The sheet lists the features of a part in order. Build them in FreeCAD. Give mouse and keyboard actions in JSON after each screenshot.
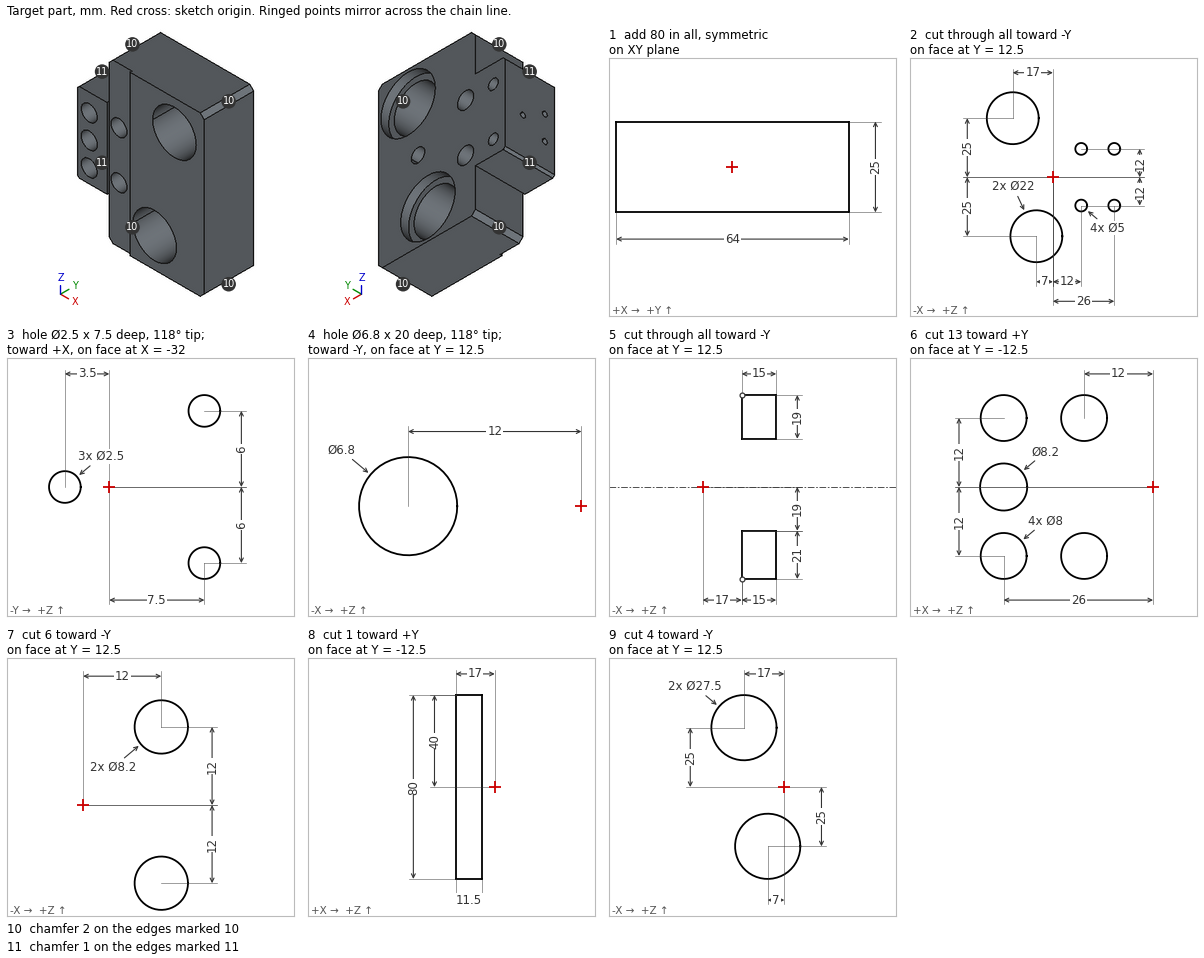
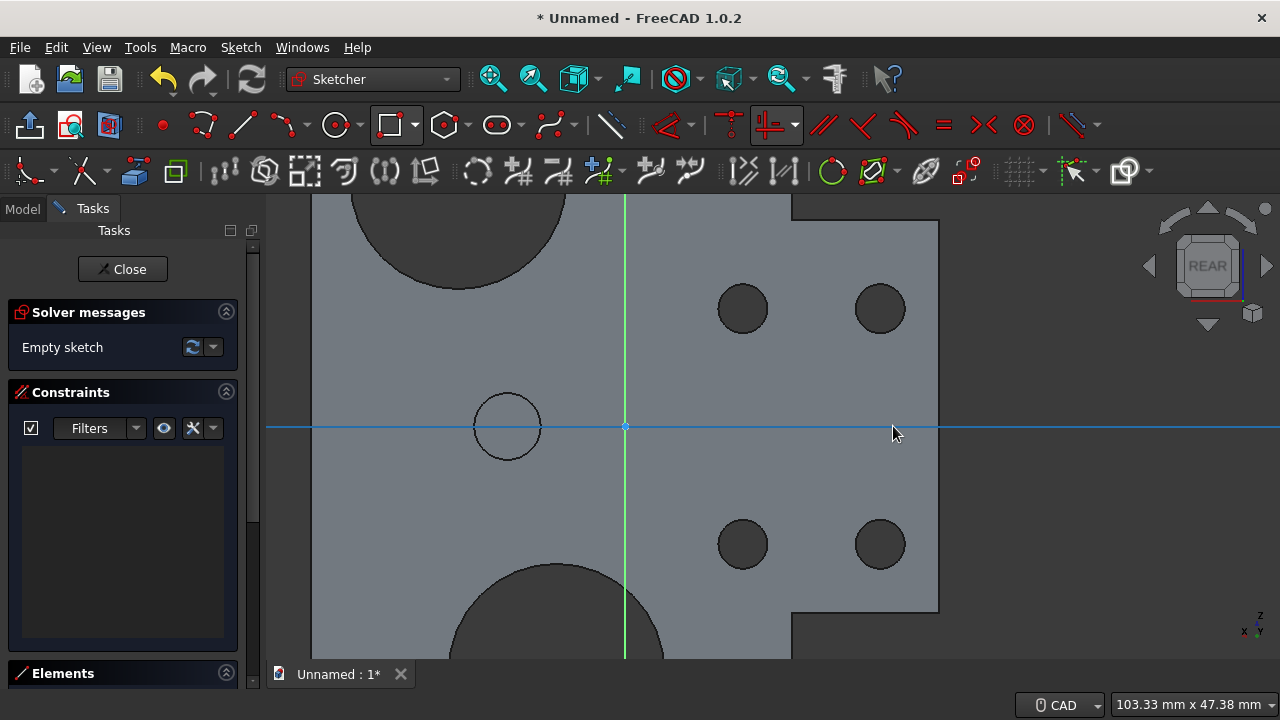
{"action": "left_click", "coordinate": [336, 126]}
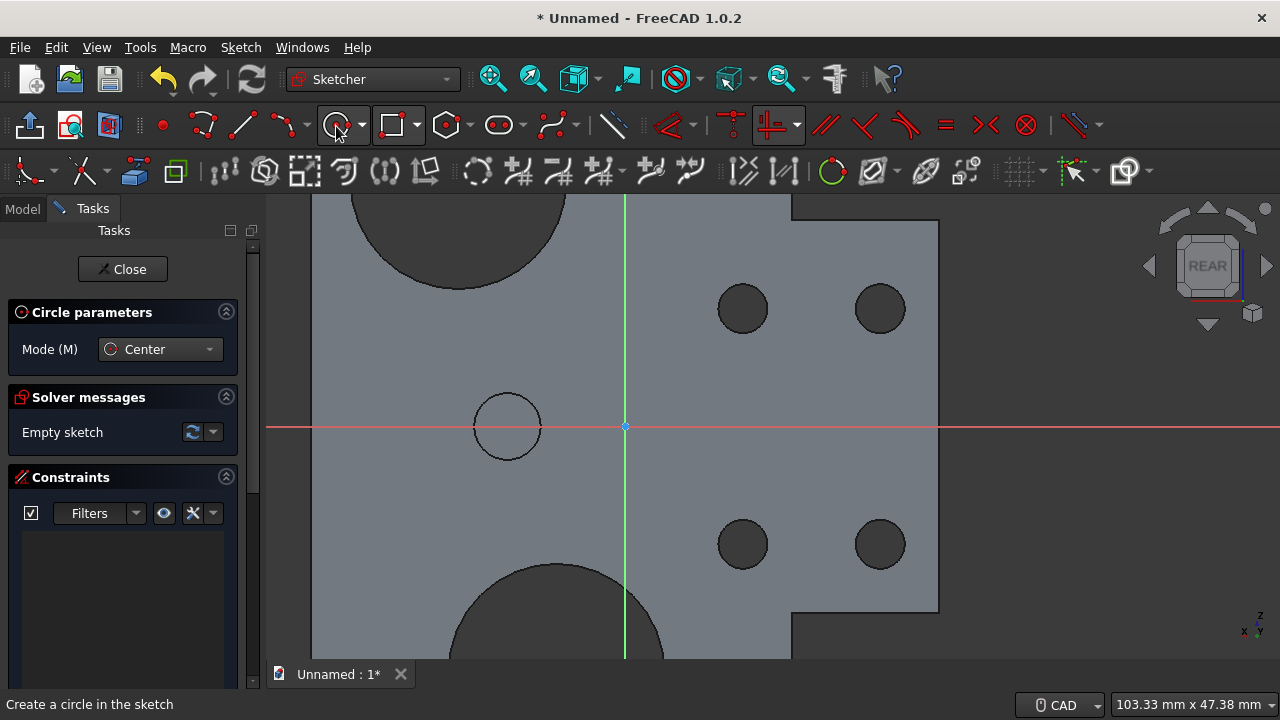
{"action": "left_click", "coordinate": [743, 309]}
{"action": "left_click", "coordinate": [771, 280]}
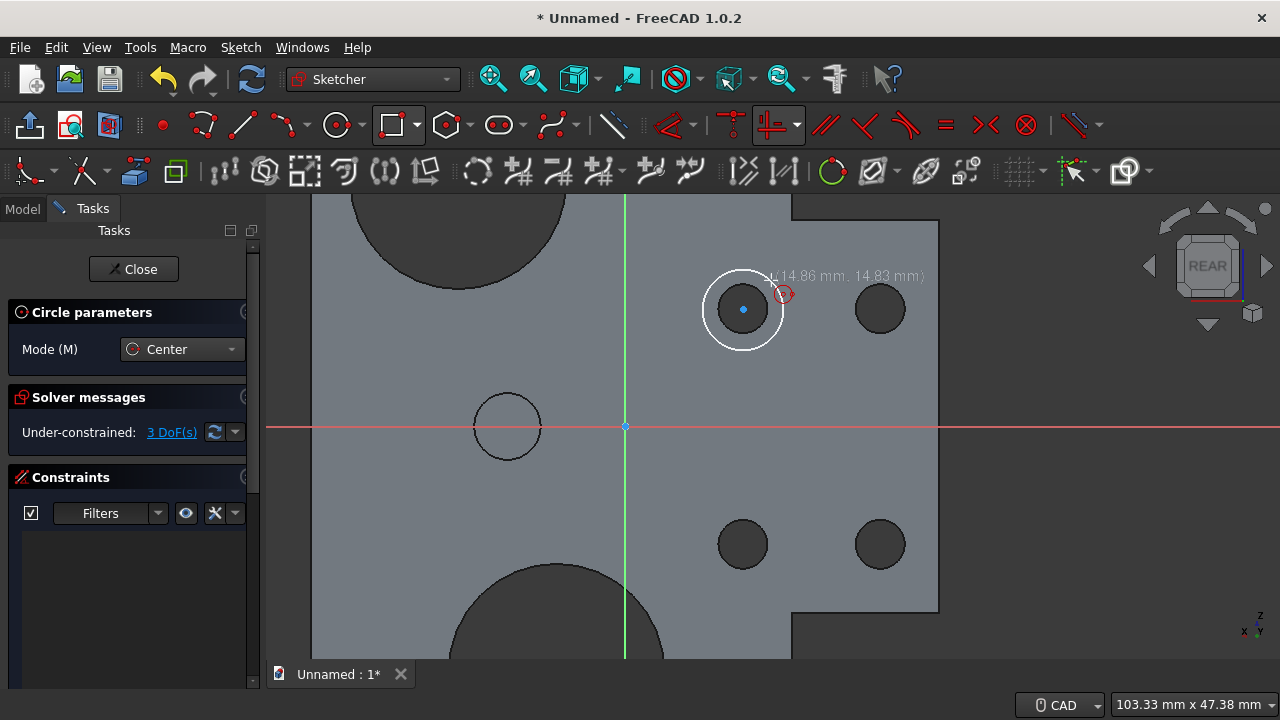
{"action": "left_click", "coordinate": [743, 544]}
{"action": "left_click", "coordinate": [771, 516]}
{"action": "key", "text": "Escape"}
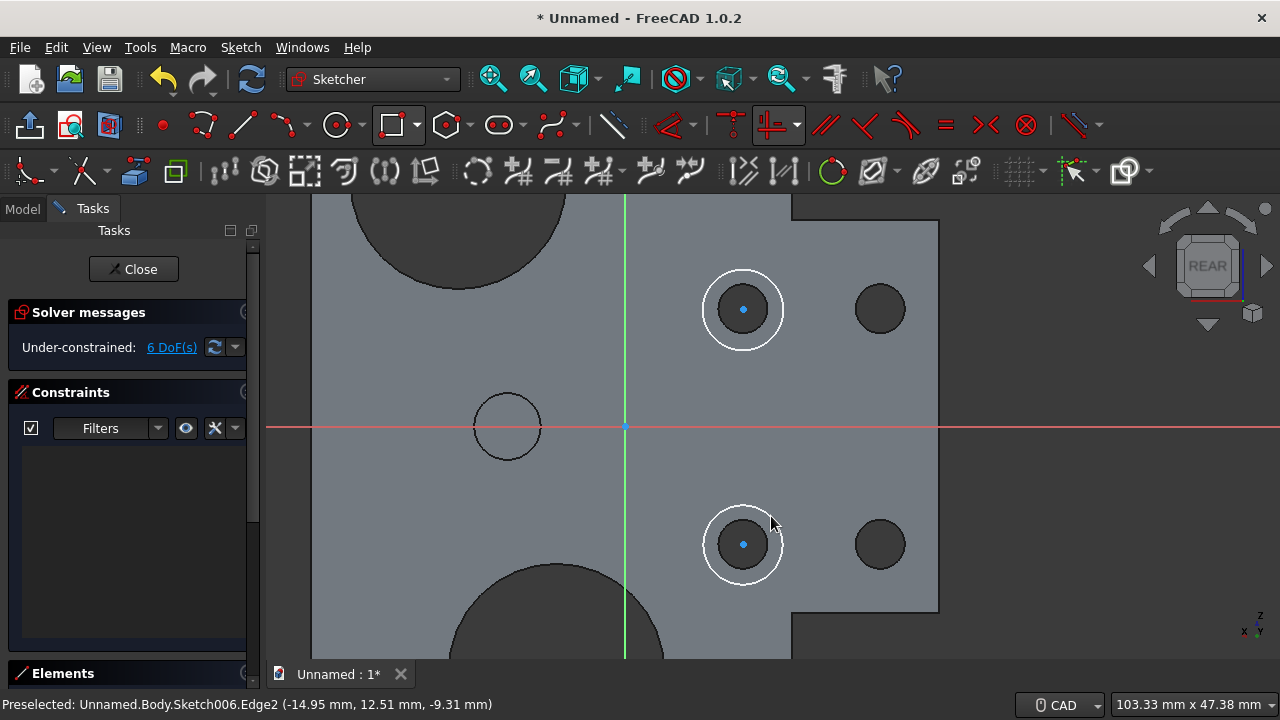
{"action": "left_click", "coordinate": [771, 281]}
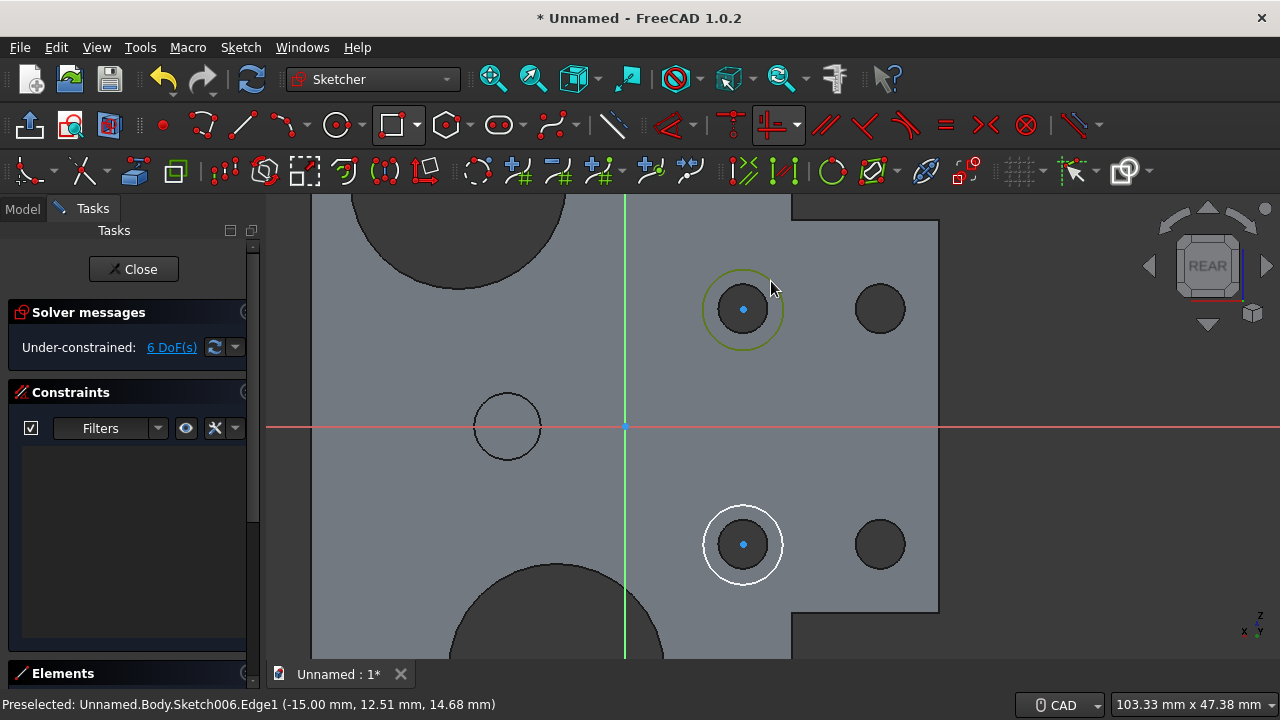
{"action": "left_click", "coordinate": [771, 517]}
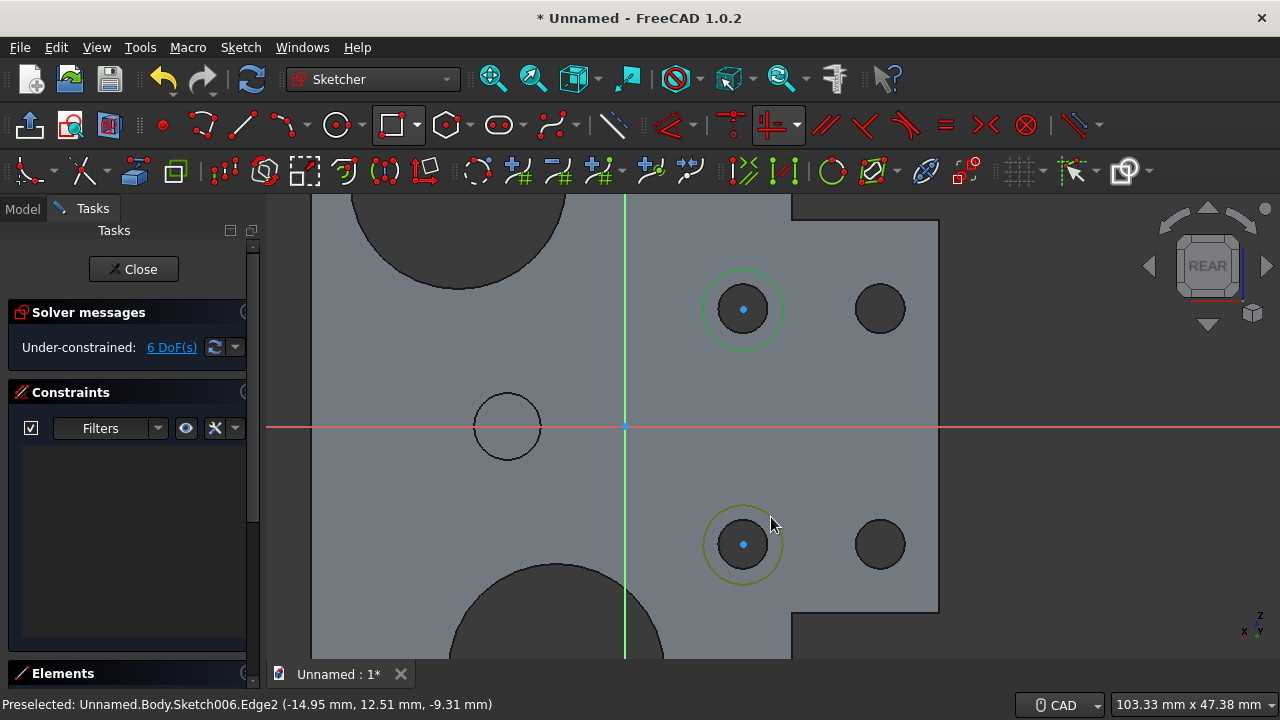
{"action": "left_click", "coordinate": [946, 126]}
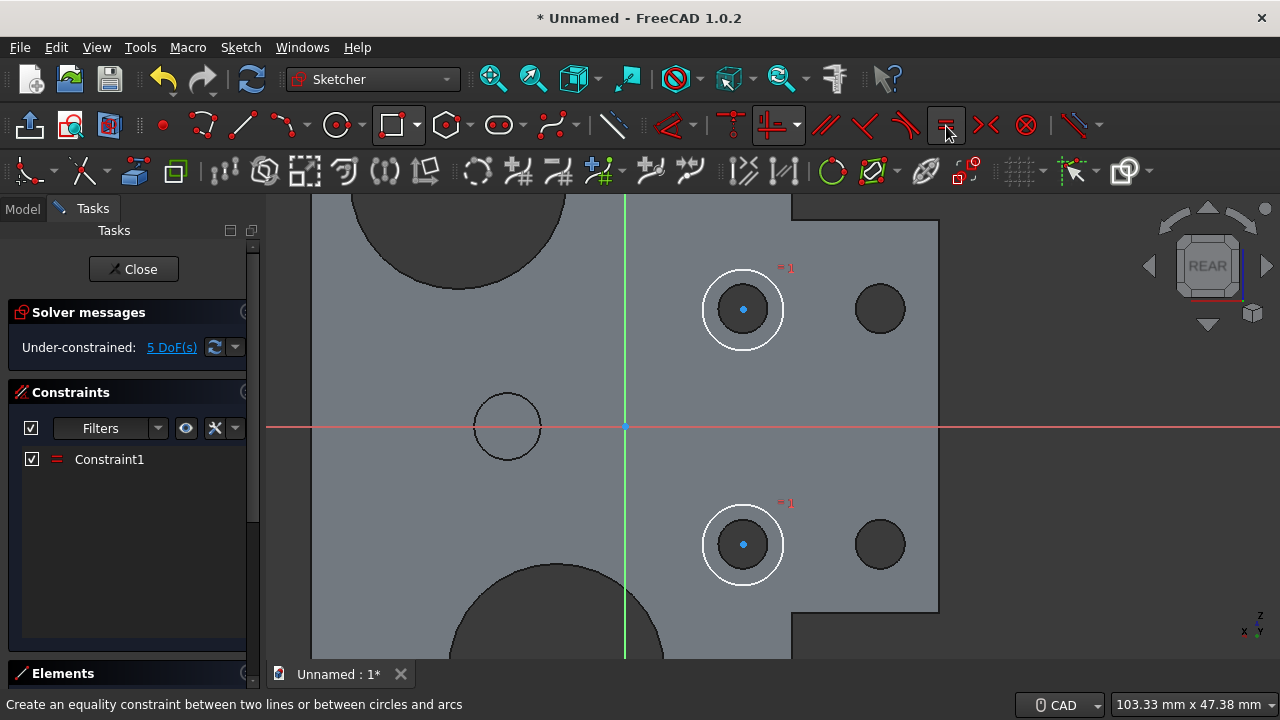
{"action": "left_click", "coordinate": [743, 310]}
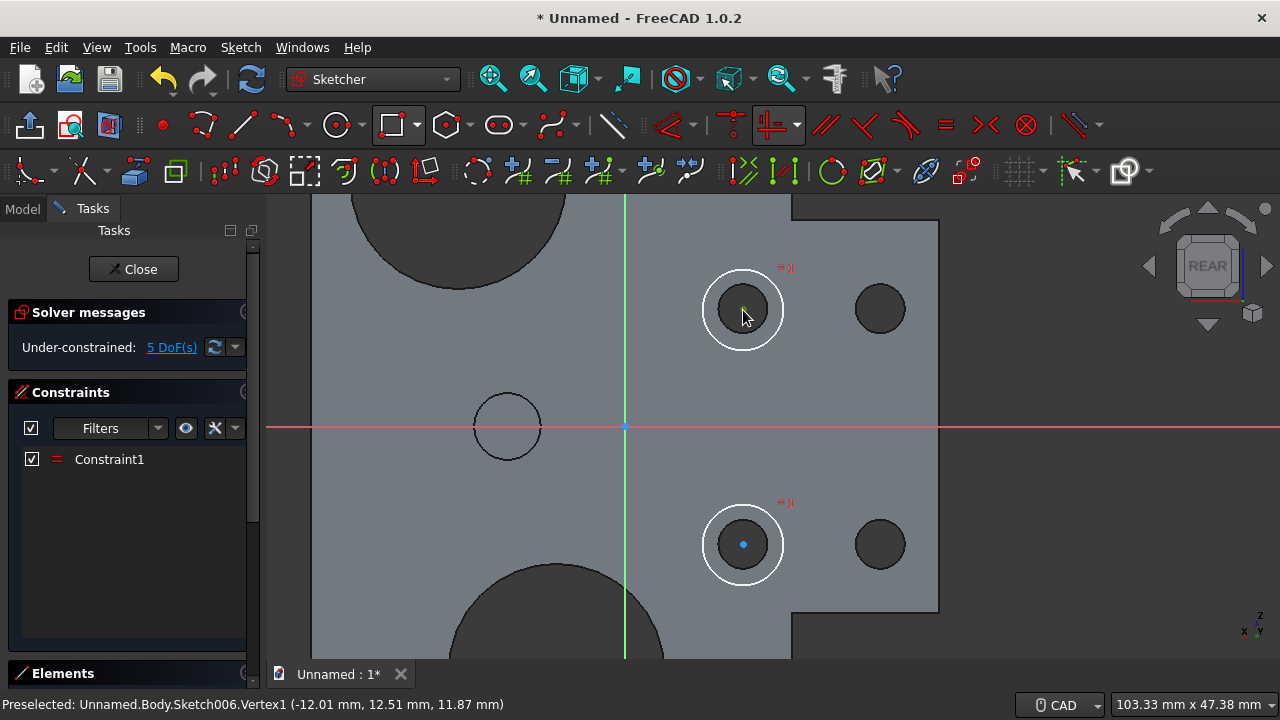
{"action": "left_click", "coordinate": [743, 545]}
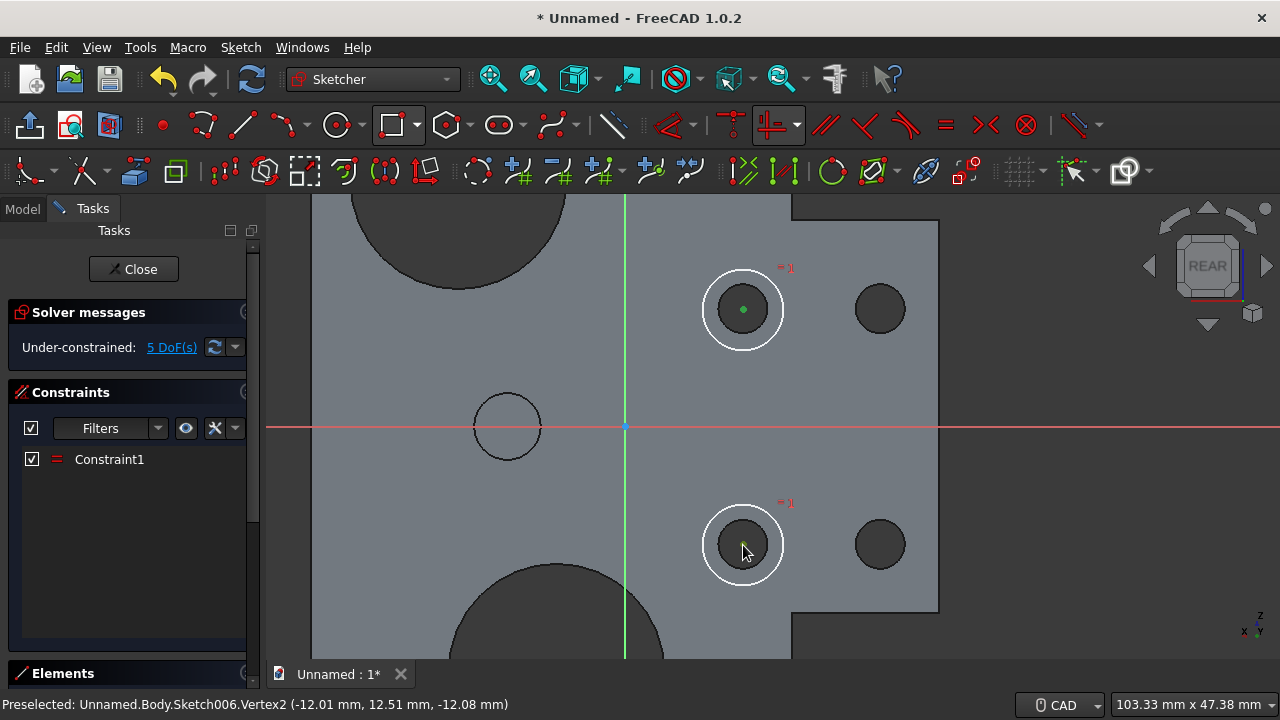
{"action": "key", "text": "v"}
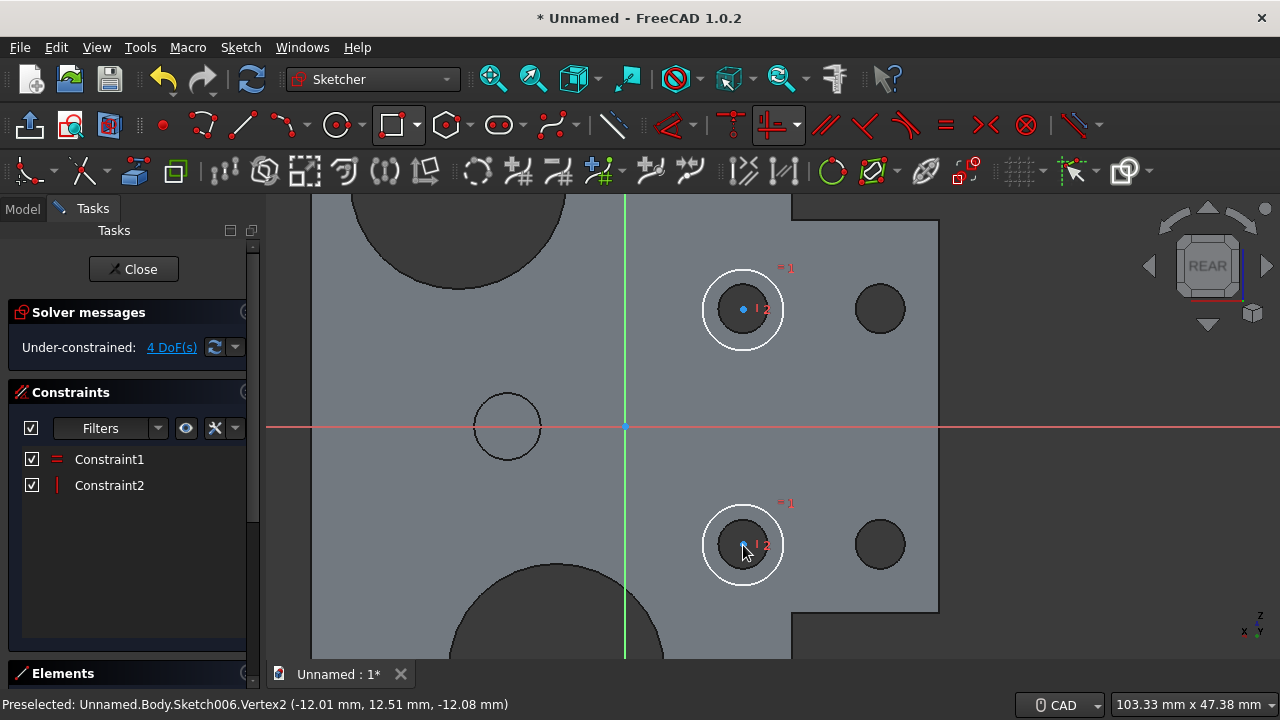
{"action": "left_click", "coordinate": [668, 126]}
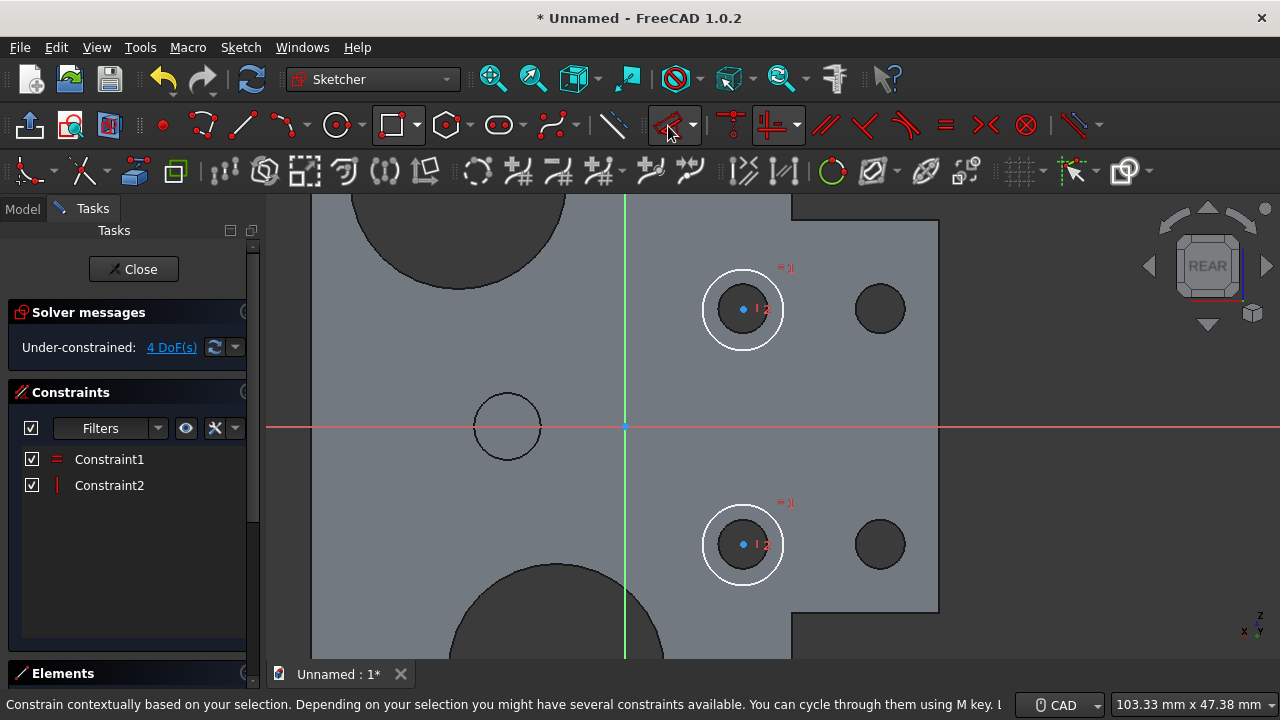
{"action": "left_click", "coordinate": [771, 281]}
{"action": "left_click", "coordinate": [793, 258]}